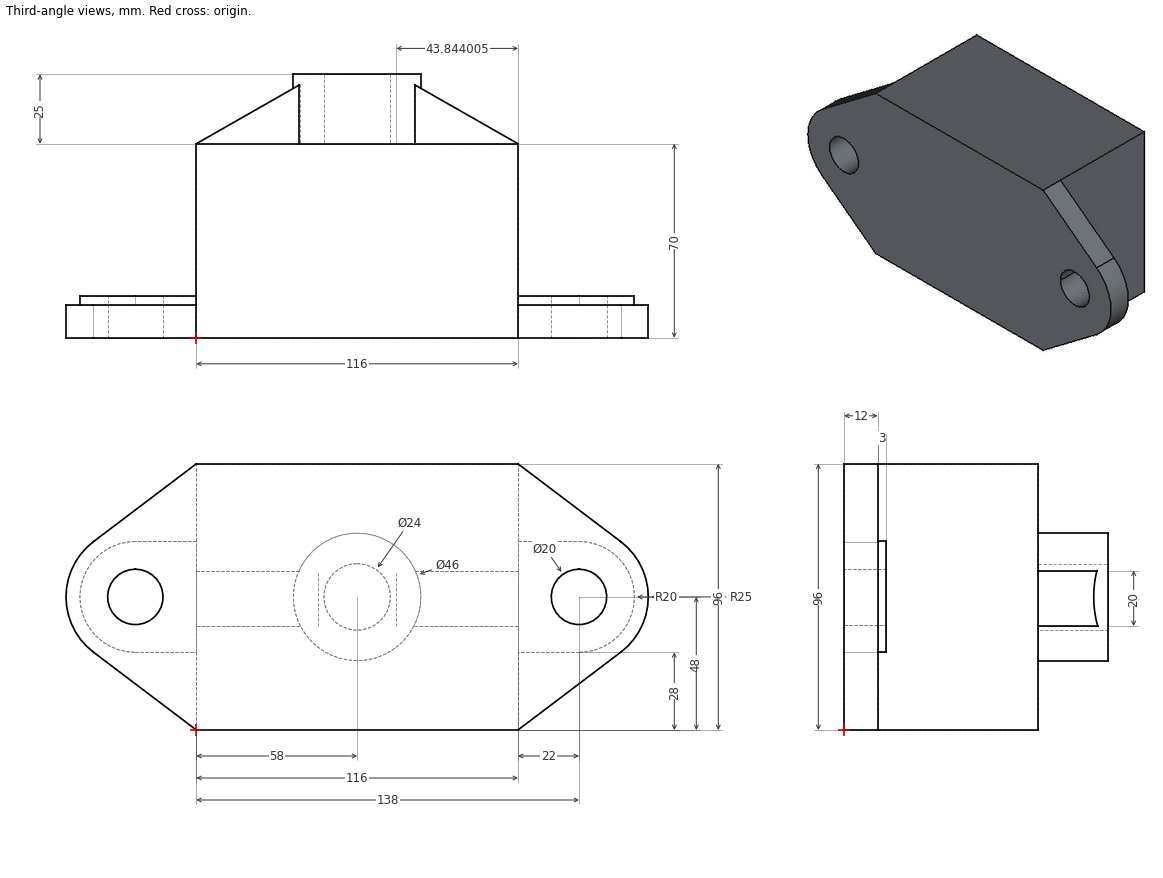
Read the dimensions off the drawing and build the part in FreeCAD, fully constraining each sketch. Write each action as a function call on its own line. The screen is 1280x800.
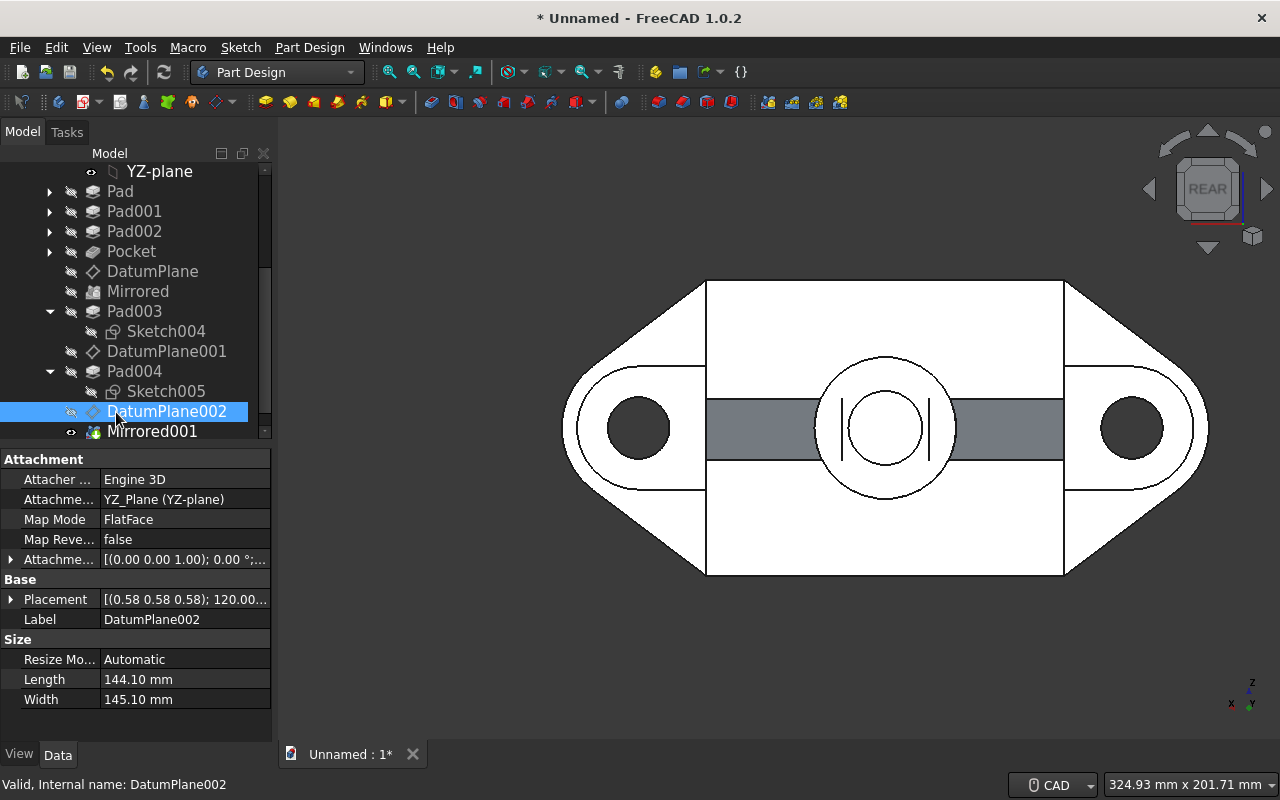
key(0)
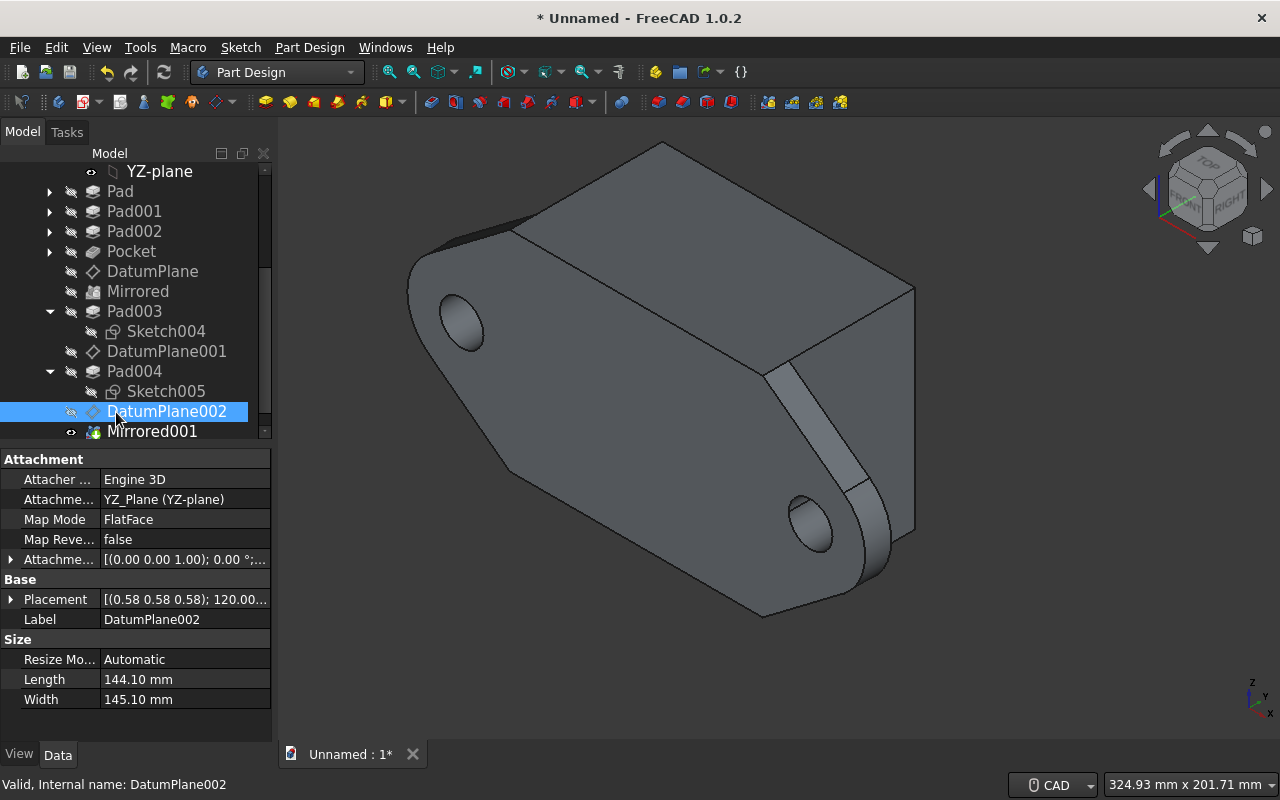
click(390, 72)